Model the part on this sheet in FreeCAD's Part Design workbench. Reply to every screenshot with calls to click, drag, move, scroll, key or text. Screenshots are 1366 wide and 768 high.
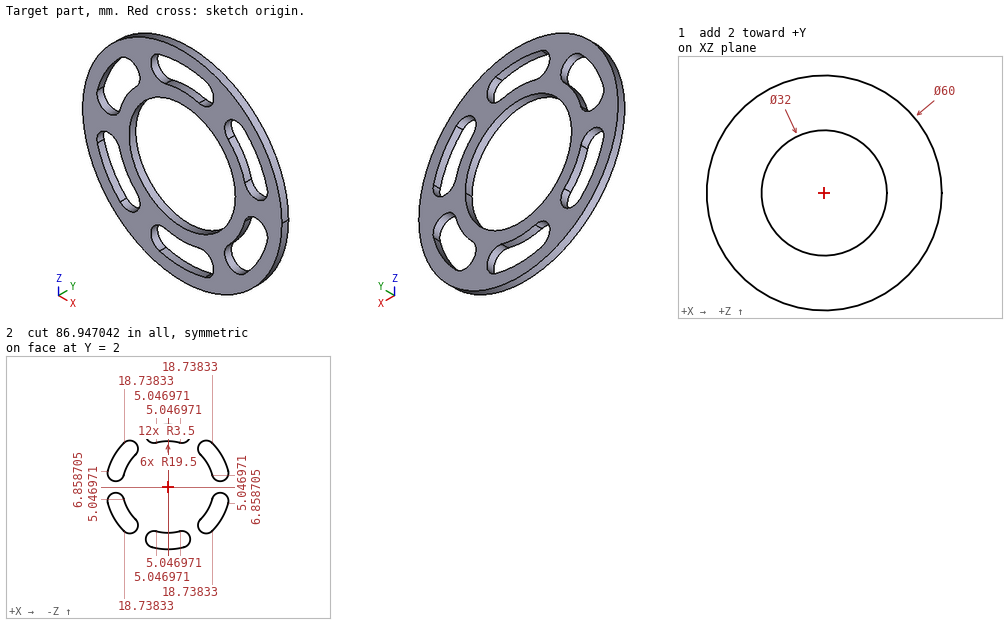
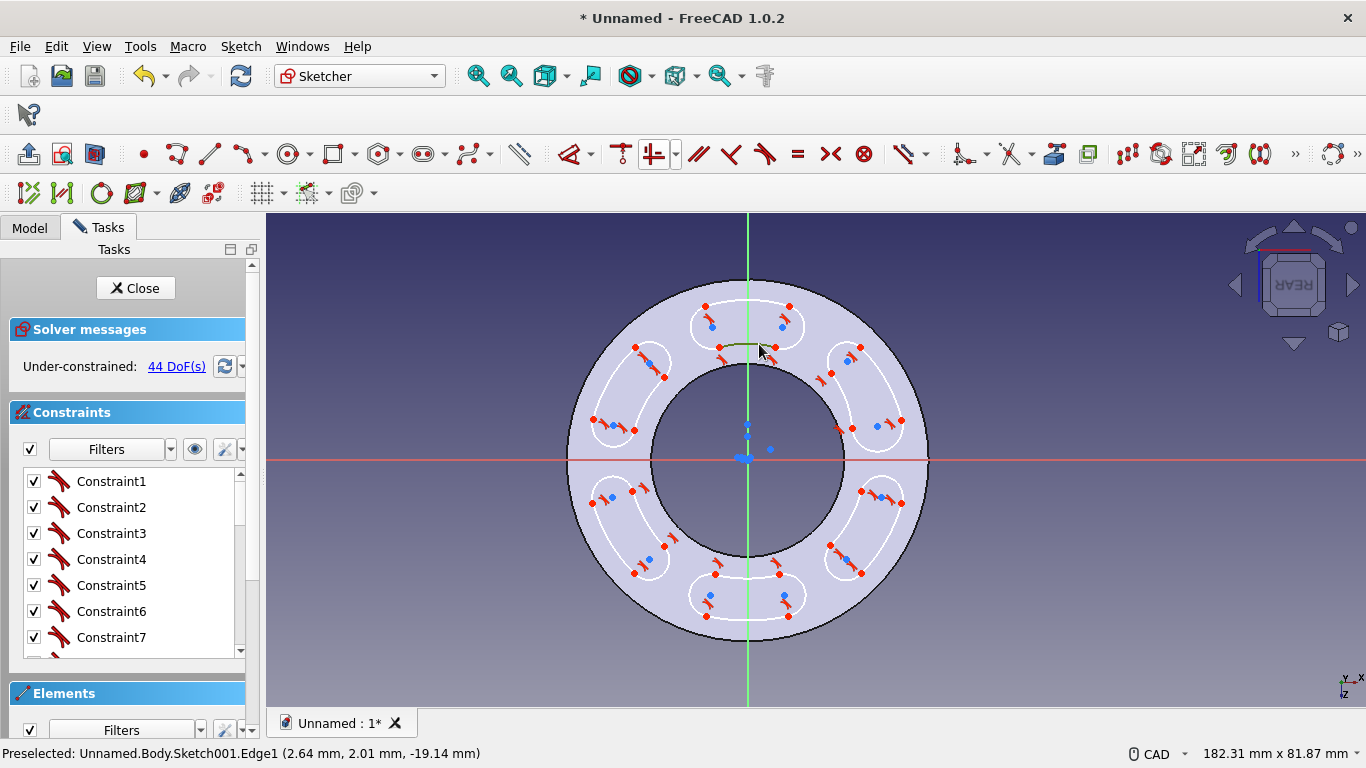
click(894, 396)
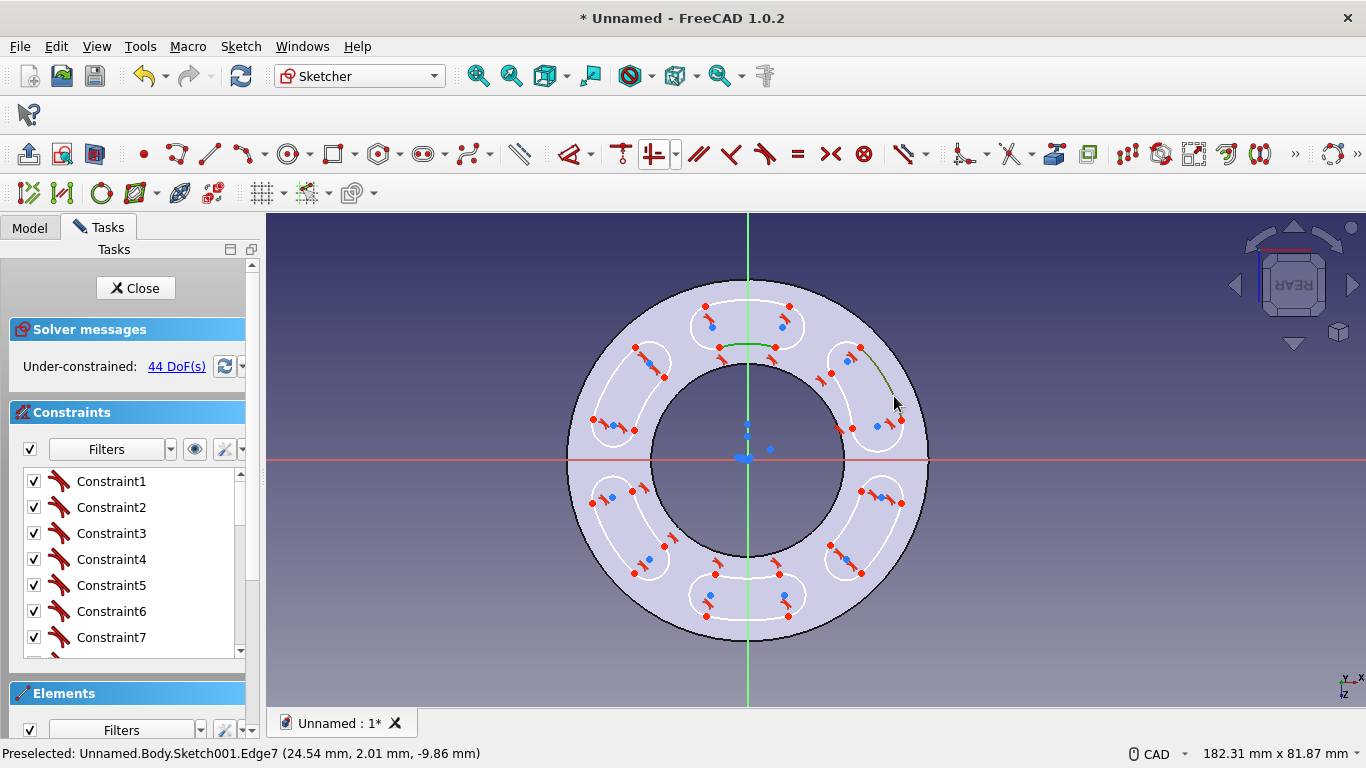
key(c)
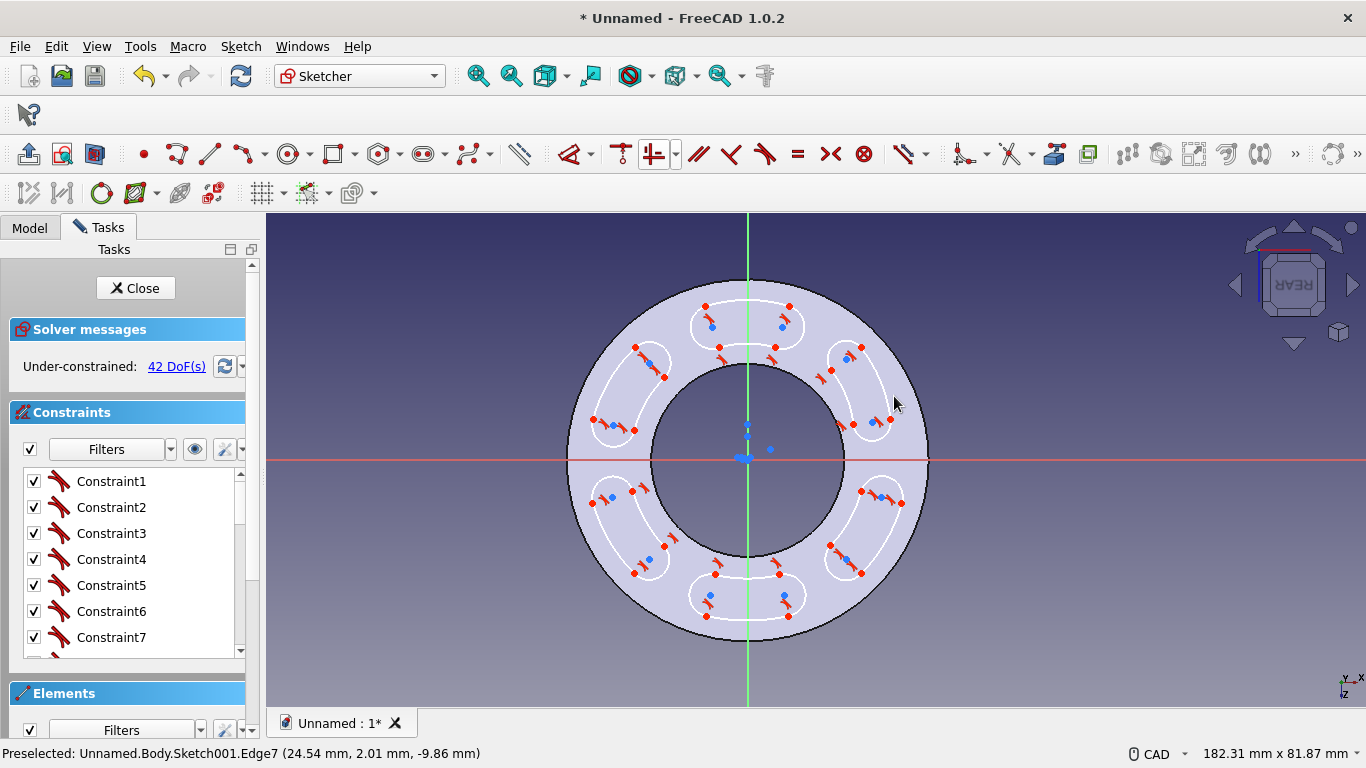
click(759, 344)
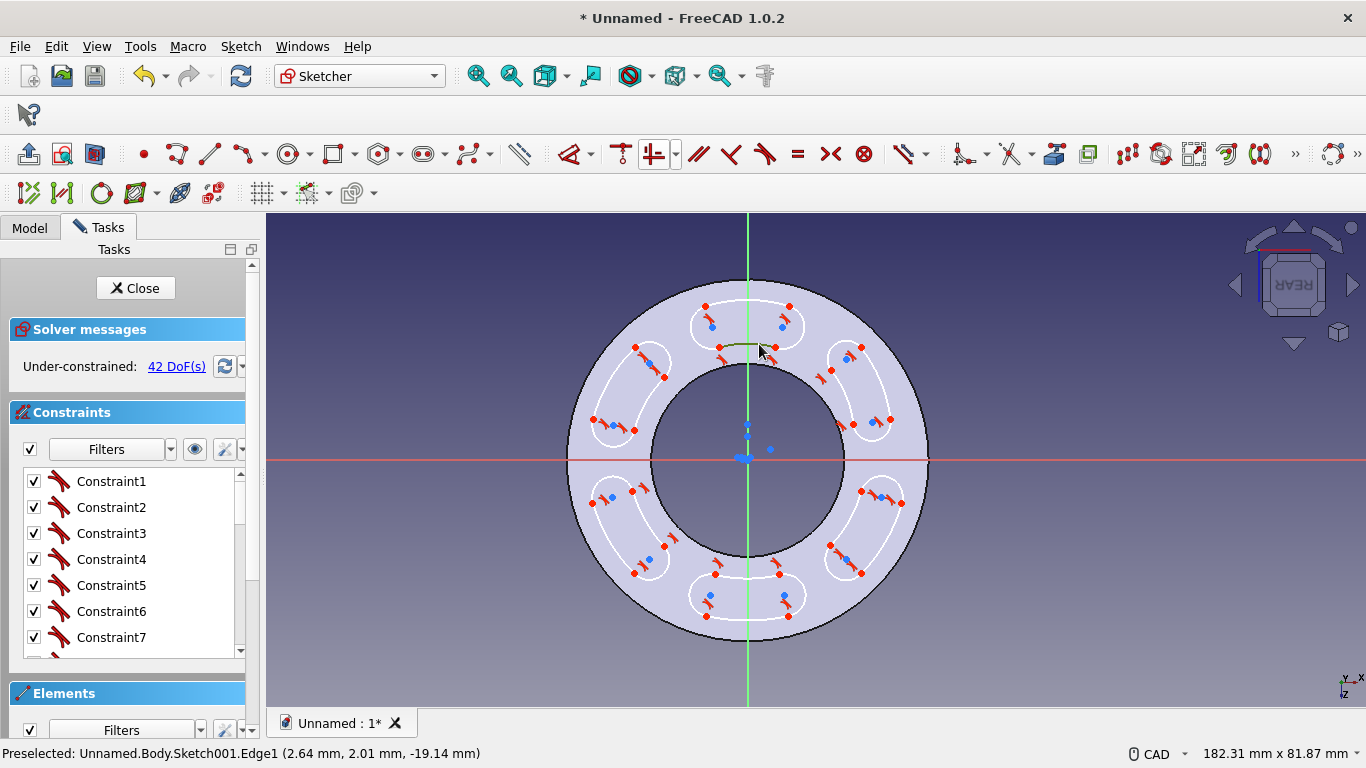
click(877, 555)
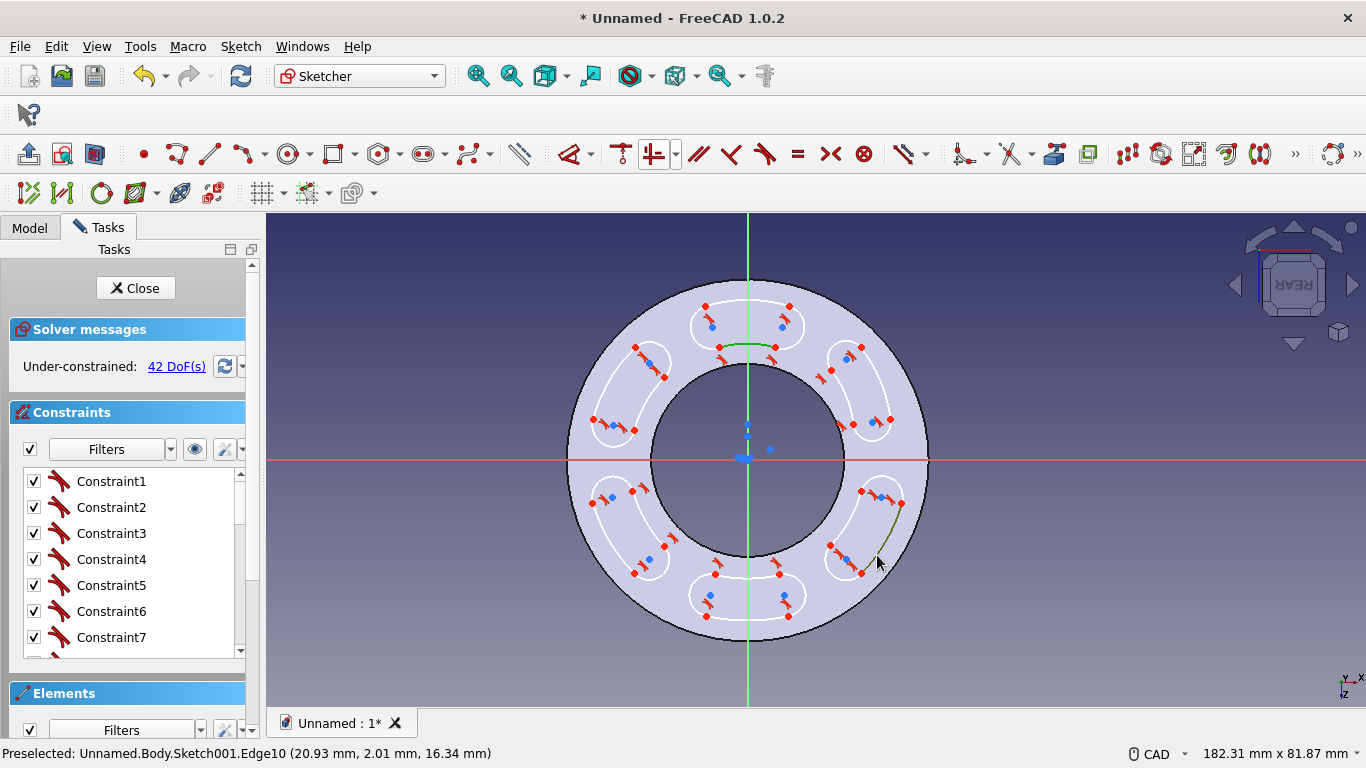
click(621, 154)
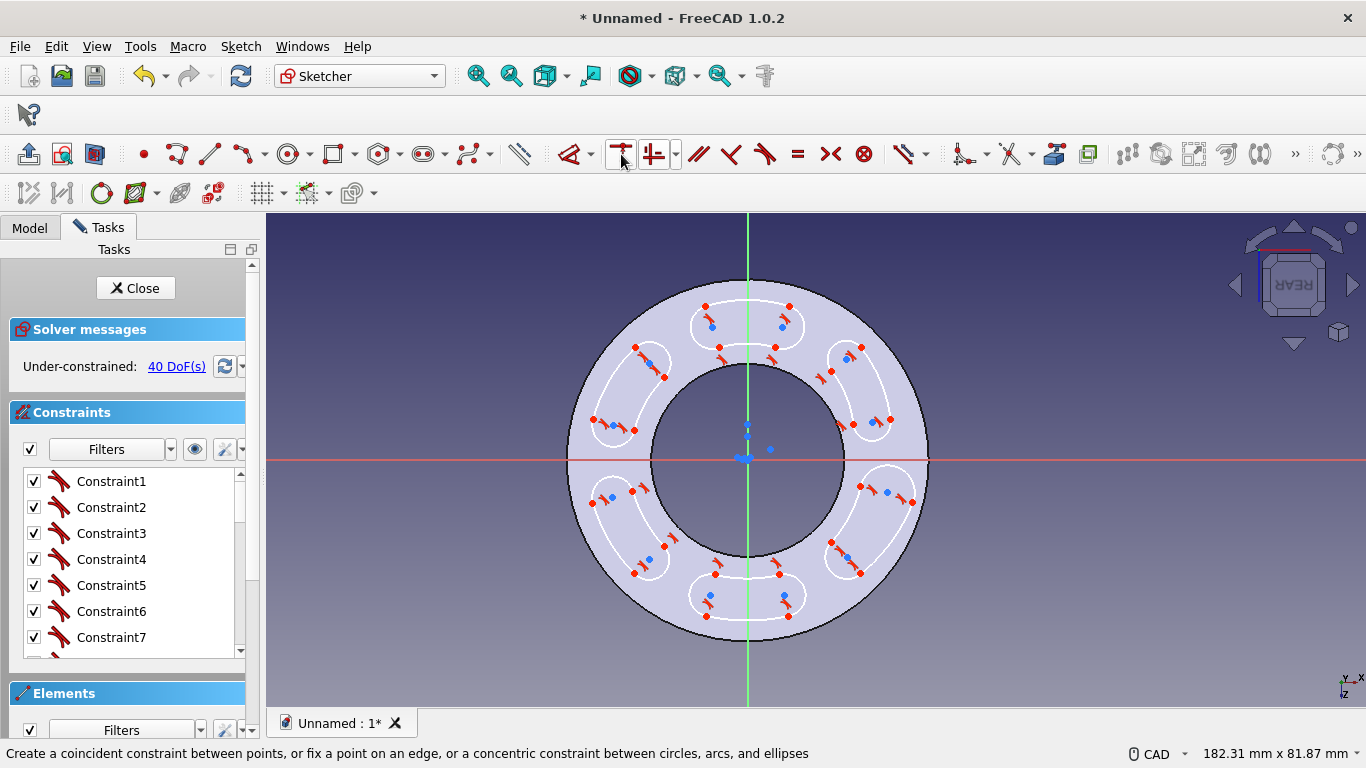
click(759, 344)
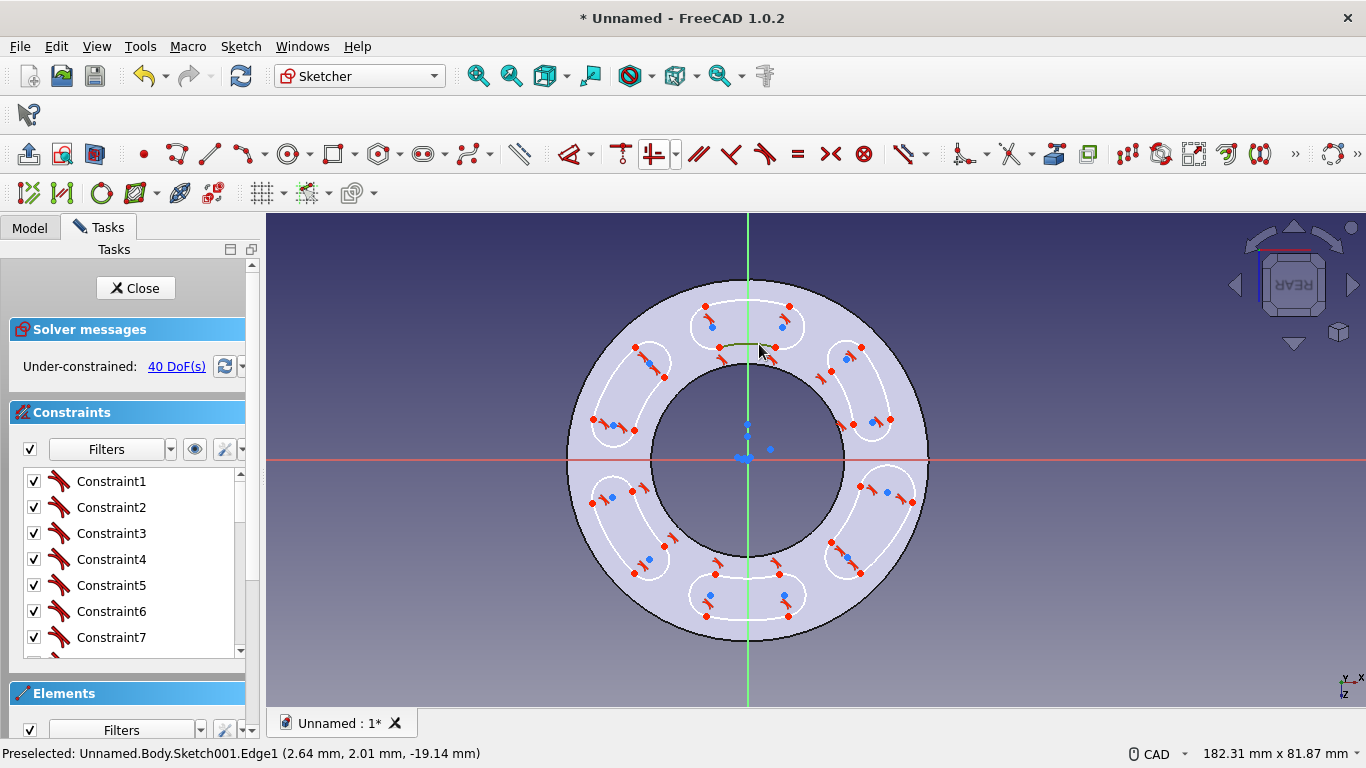
click(843, 527)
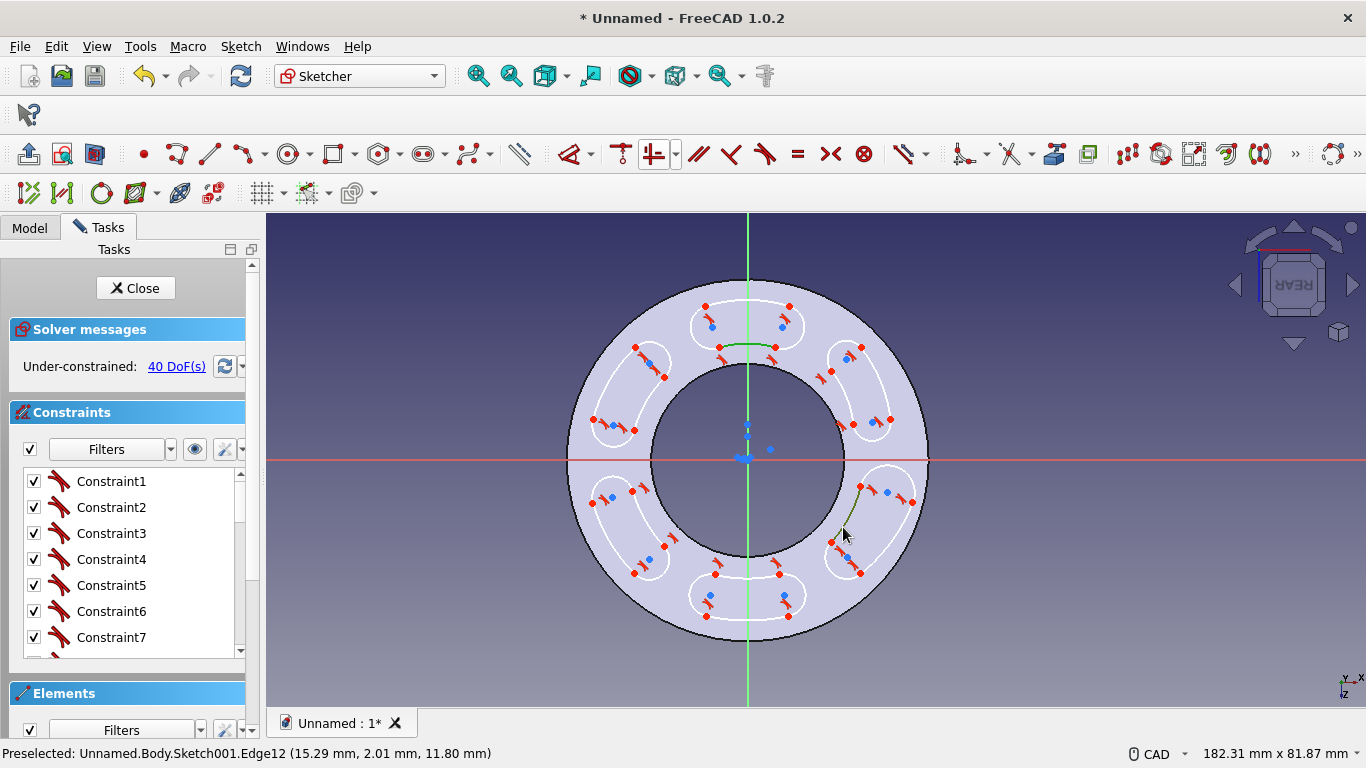
click(621, 154)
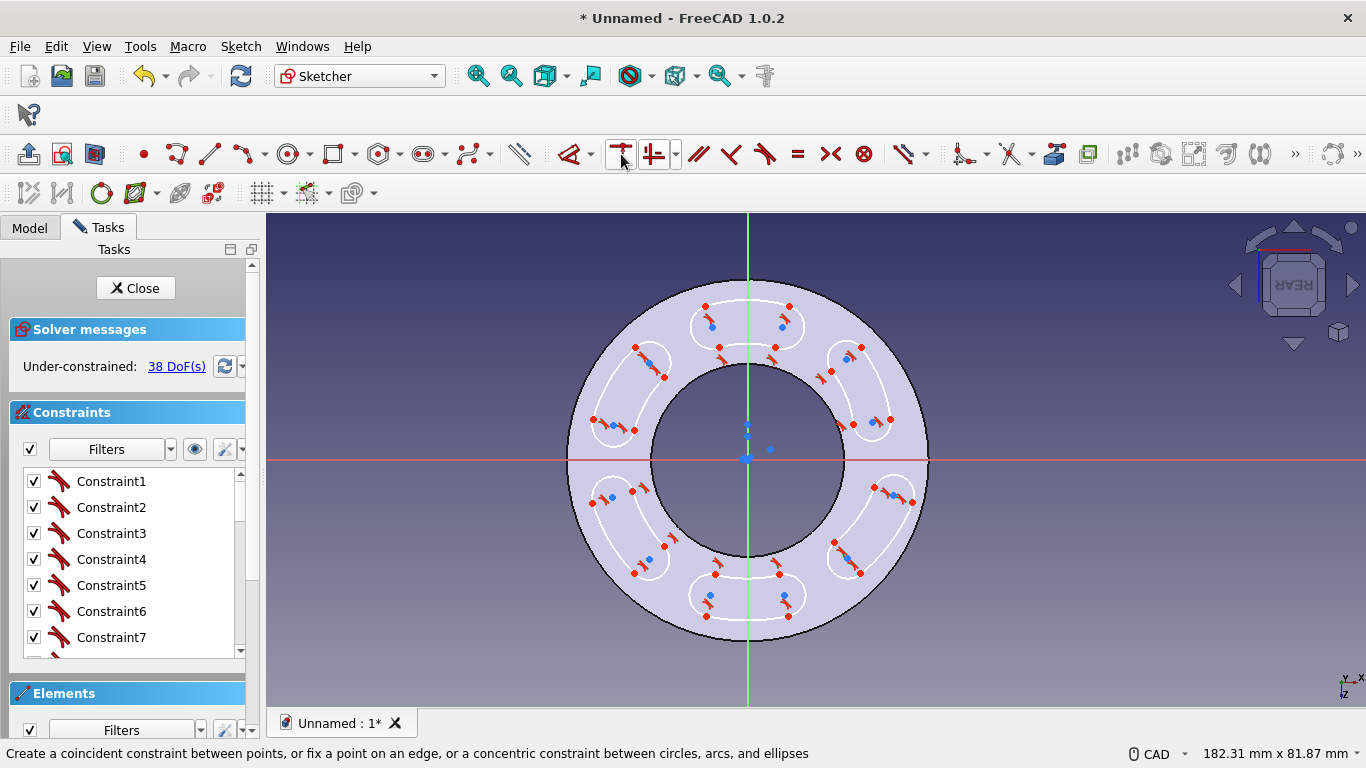
click(759, 344)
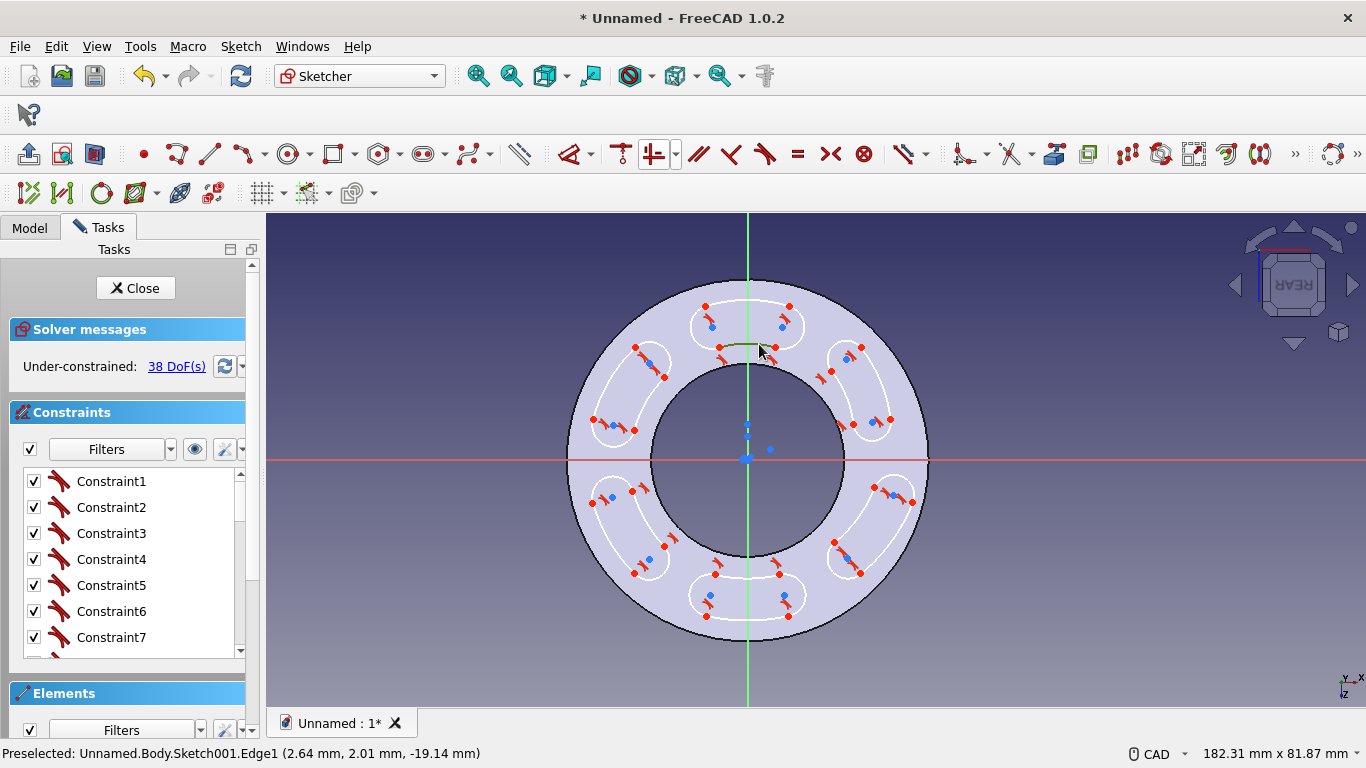
click(735, 578)